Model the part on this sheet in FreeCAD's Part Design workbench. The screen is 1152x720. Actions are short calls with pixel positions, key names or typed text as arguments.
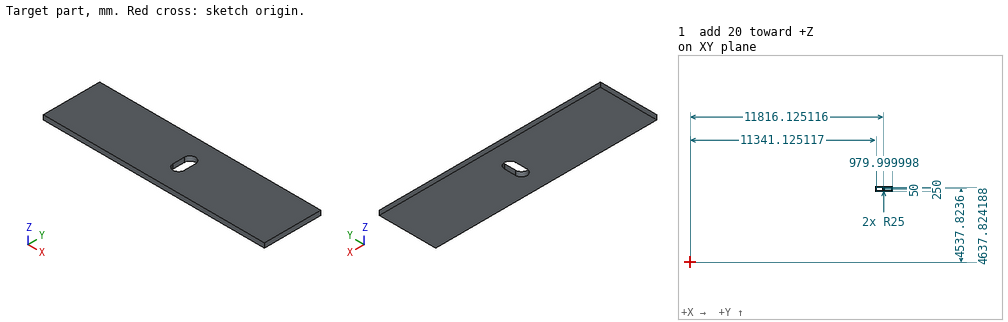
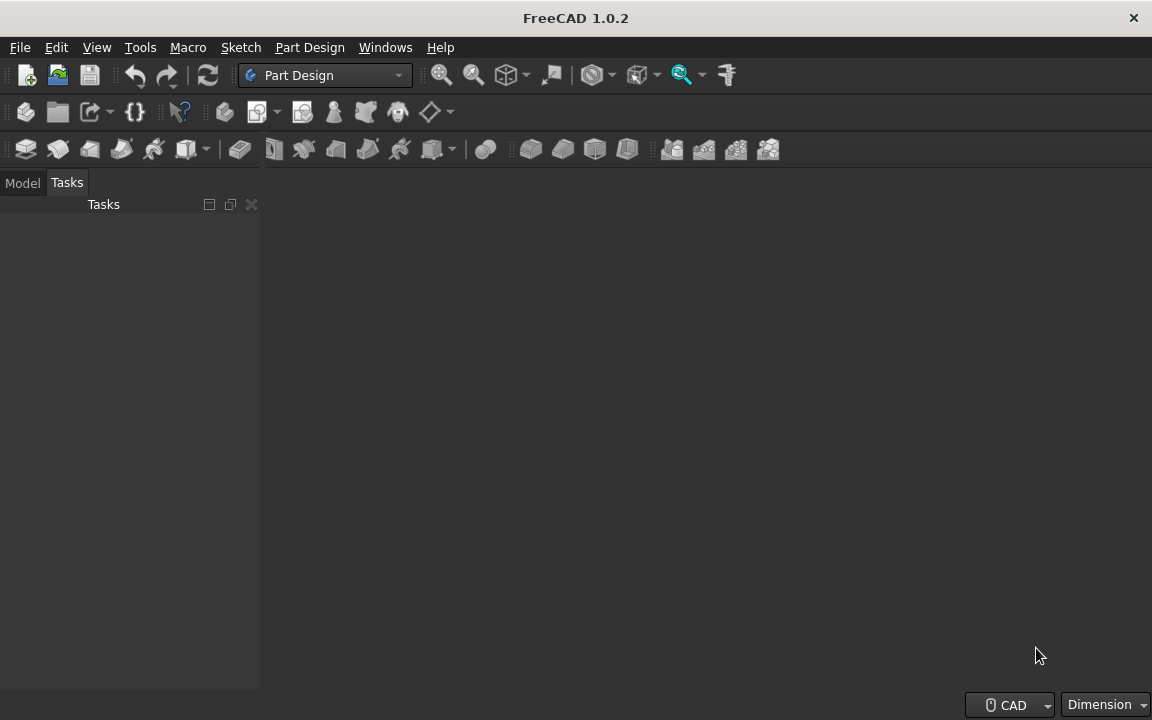
key(ctrl+n)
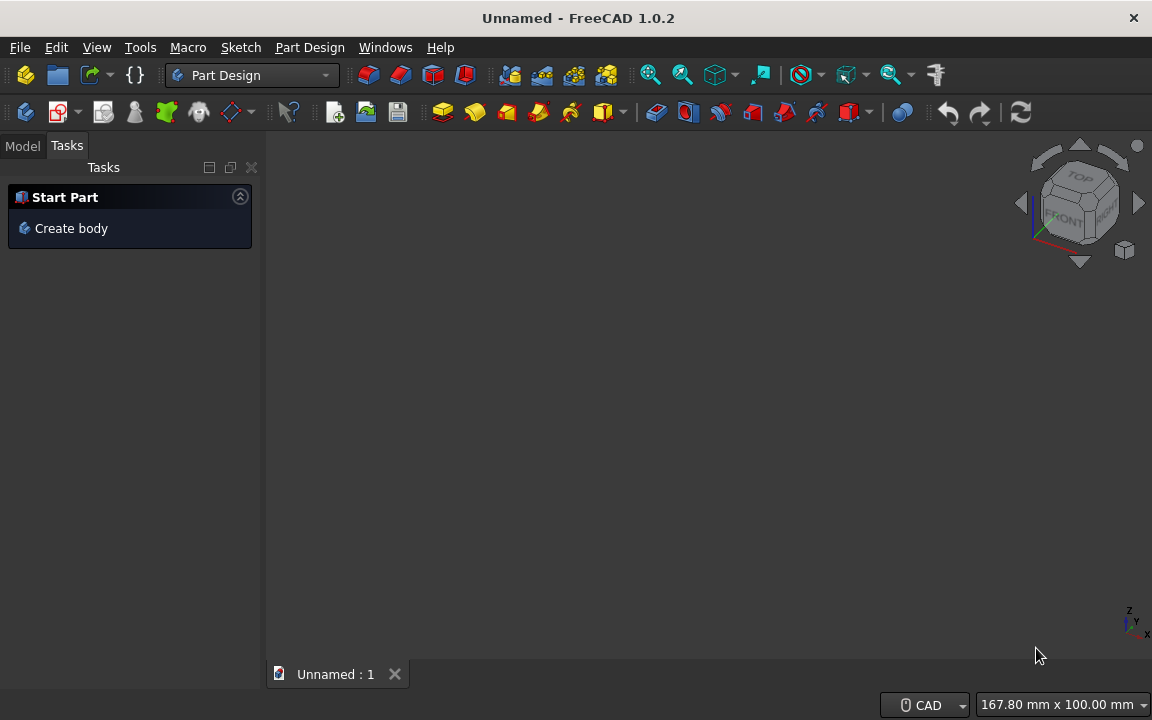
click(58, 112)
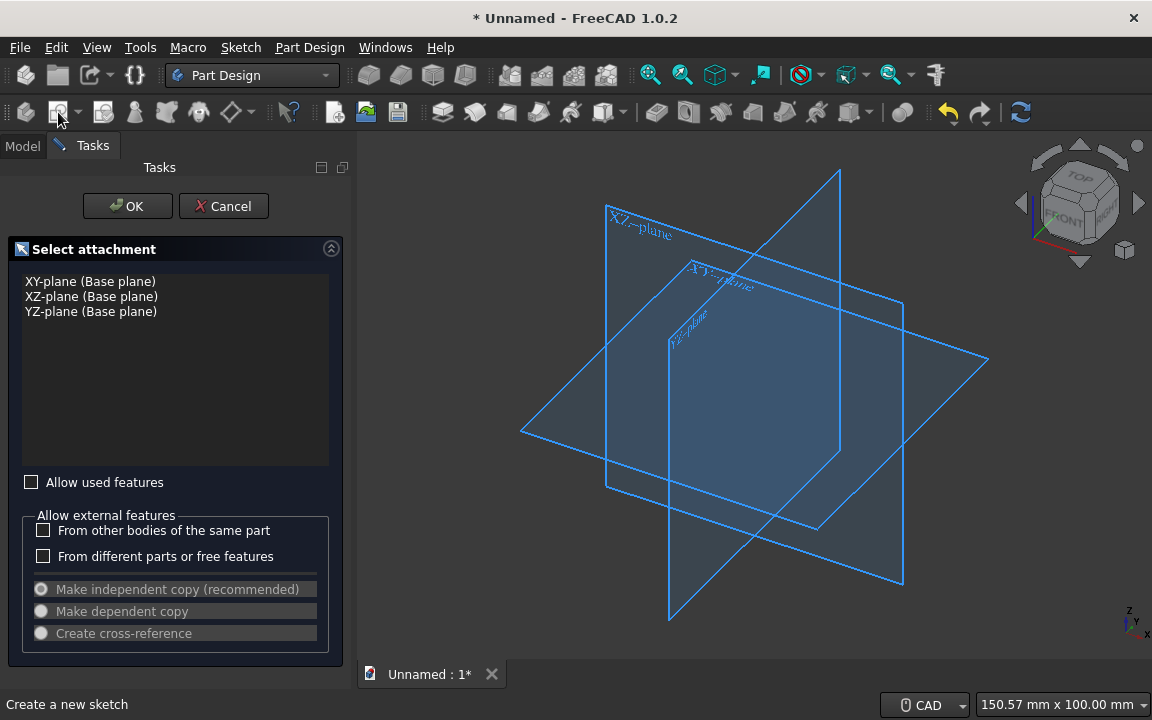
click(82, 282)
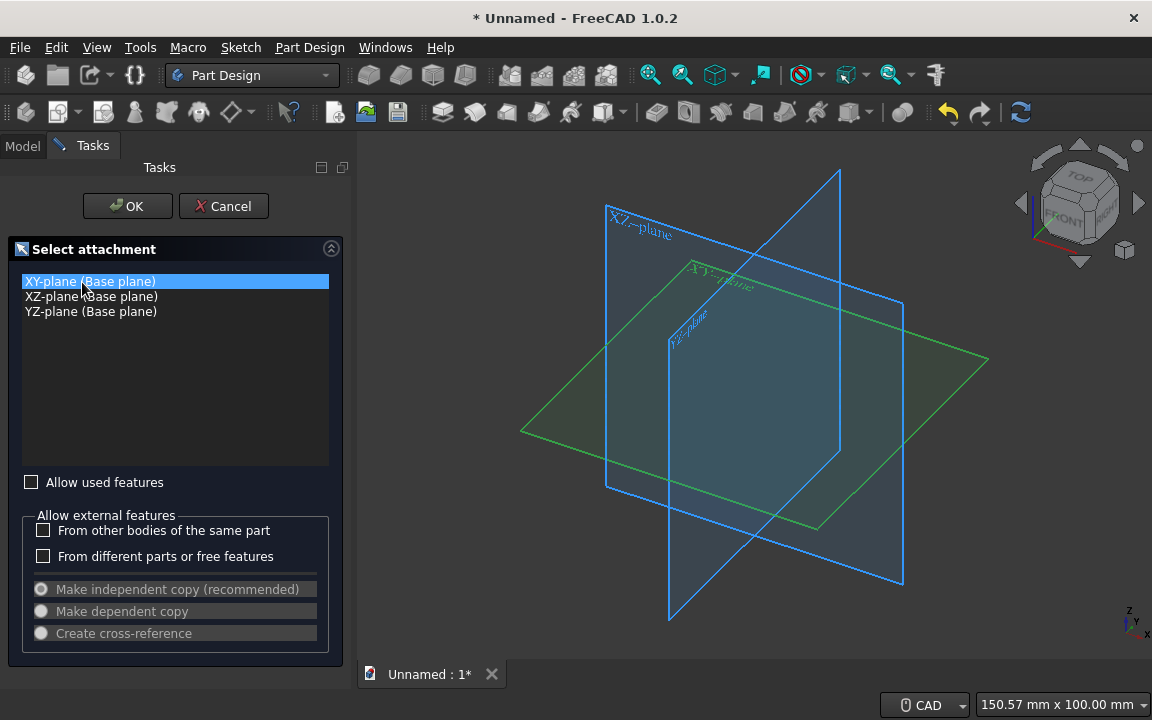
click(128, 206)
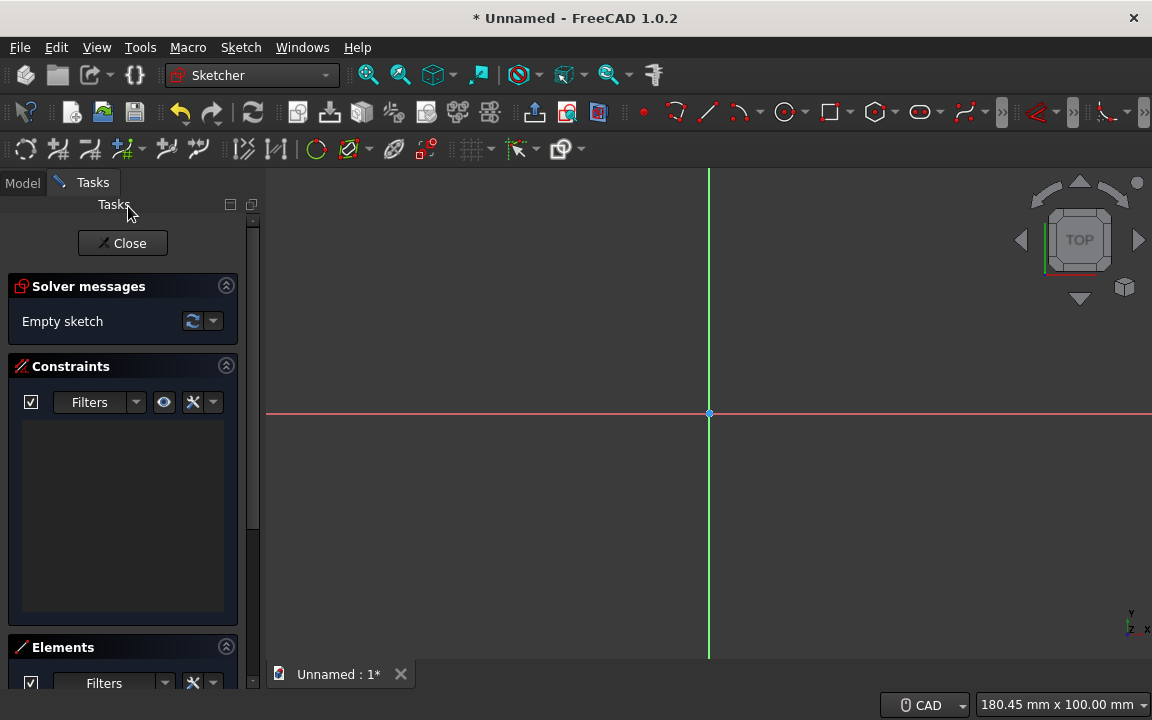
scroll(640, 414, down, 11)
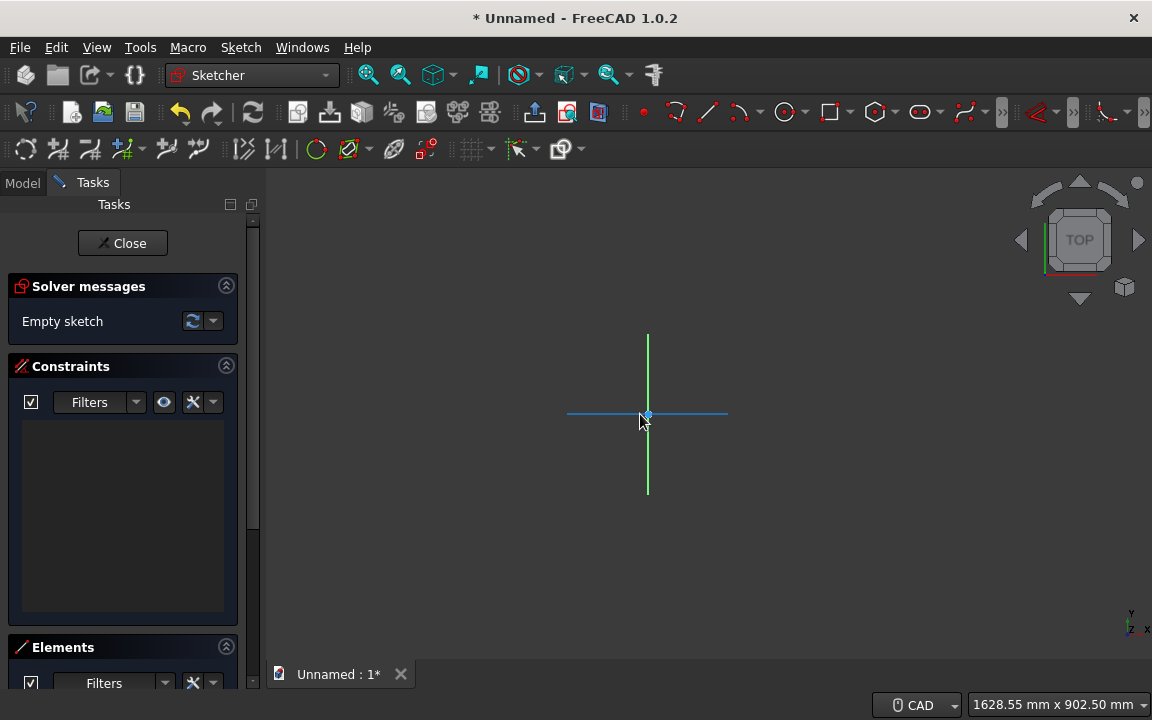
scroll(640, 414, down, 5)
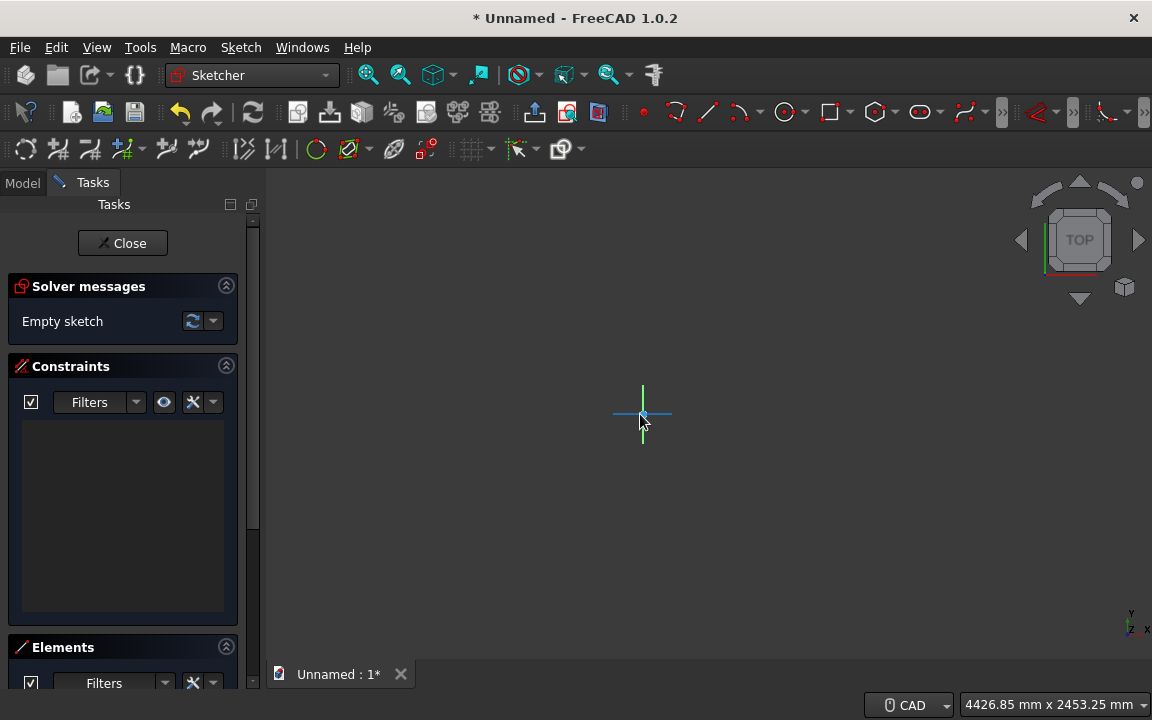
scroll(640, 414, down, 5)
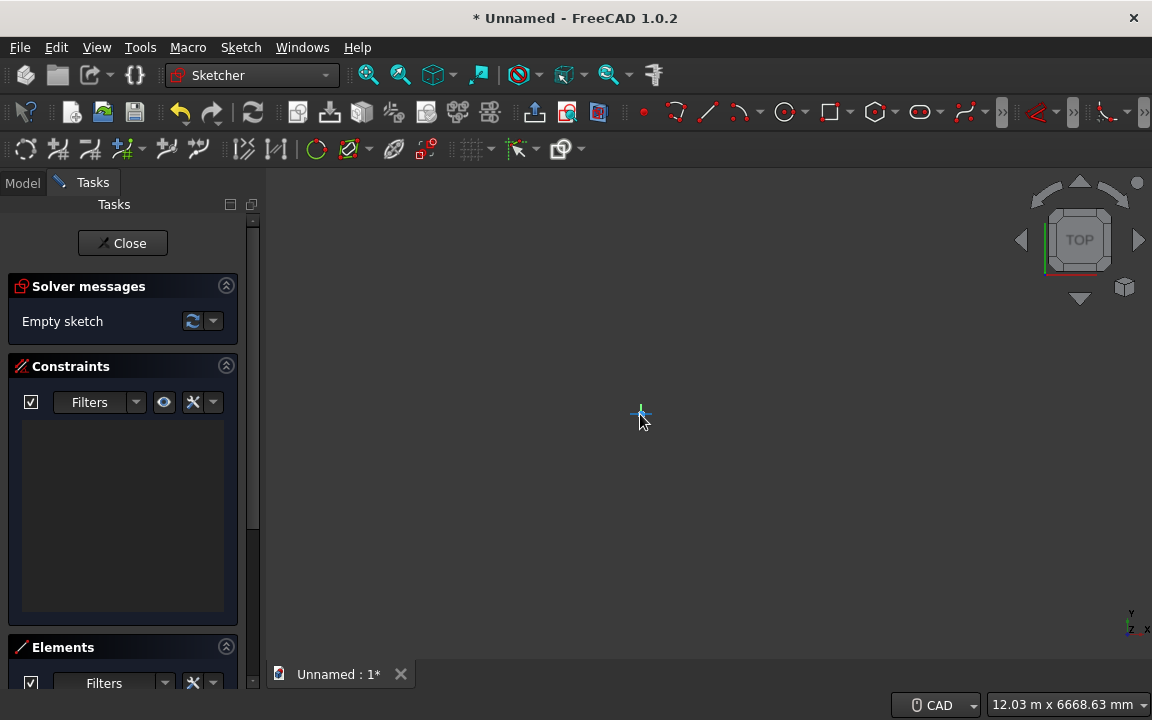
scroll(640, 414, down, 5)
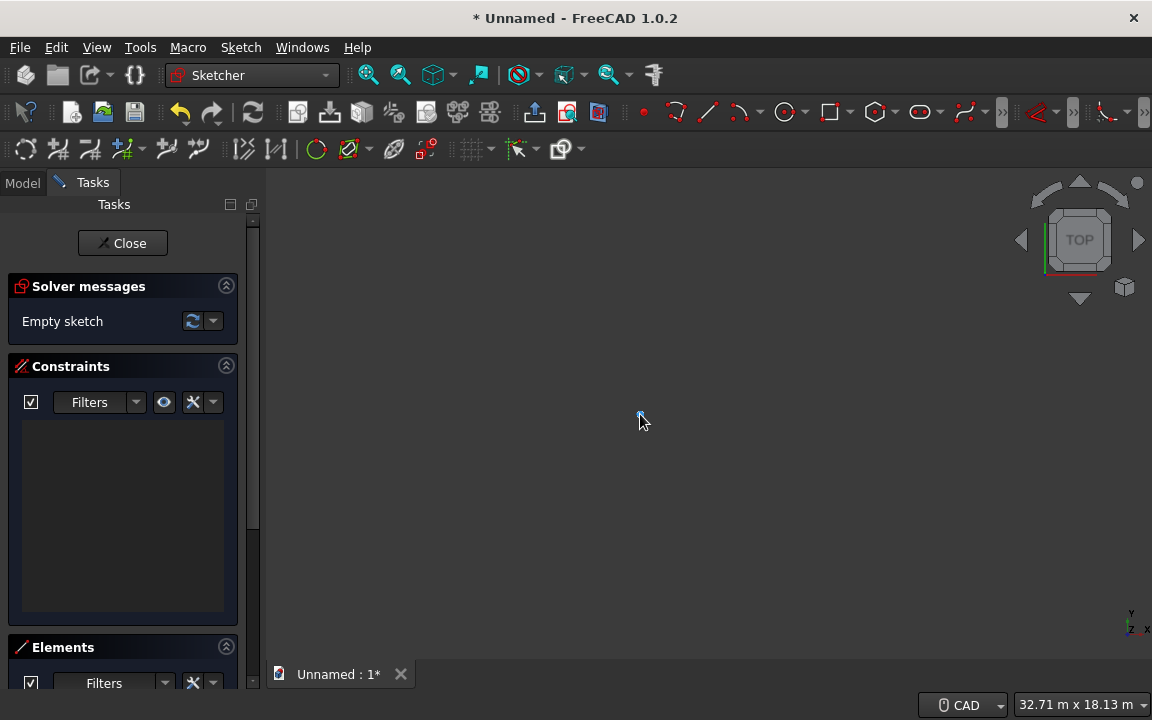
scroll(978, 286, up, 15)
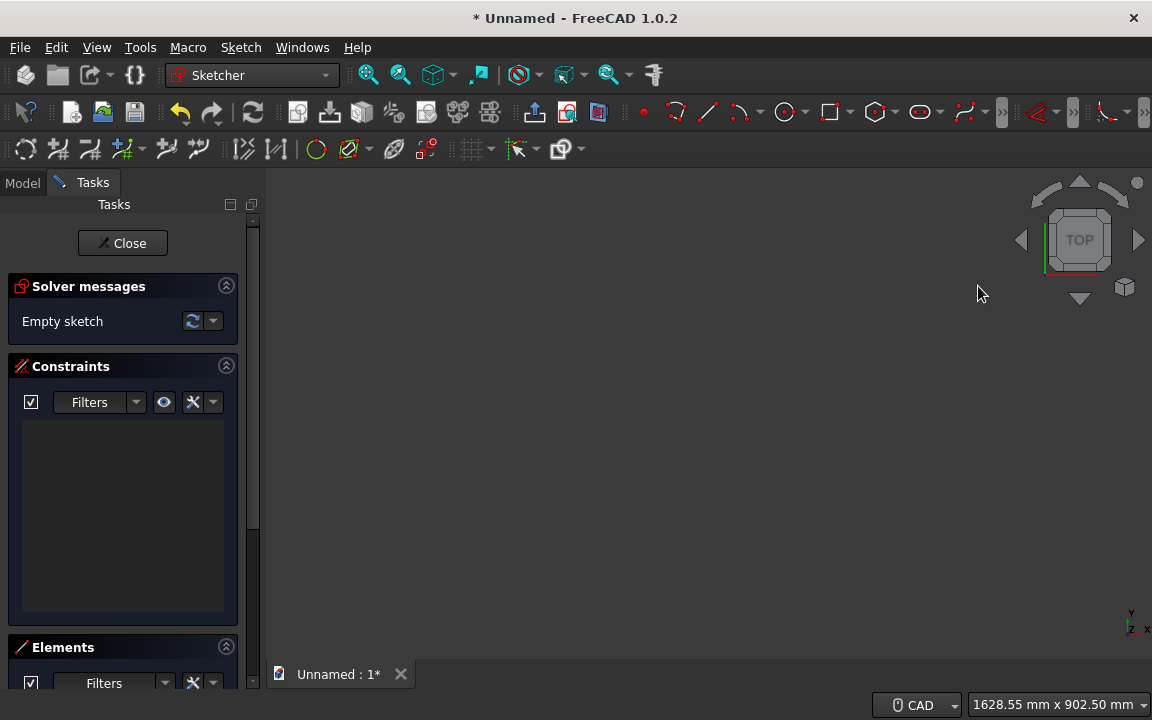
key(g)
key(r)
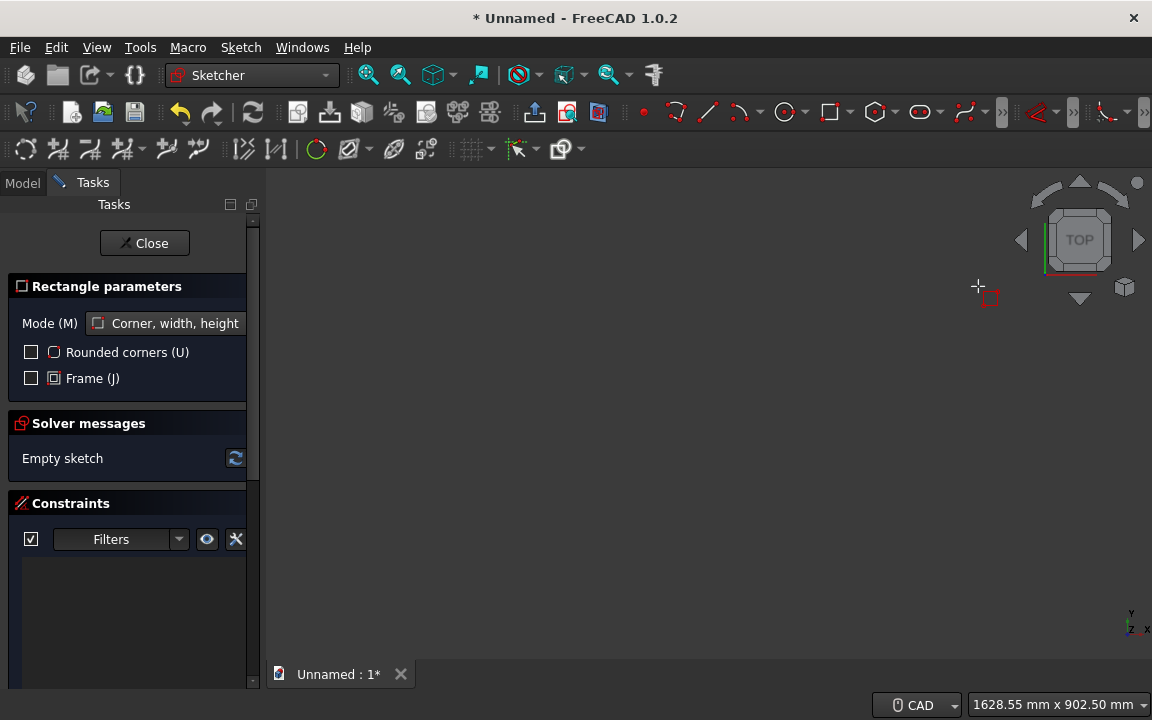
click(360, 339)
click(893, 475)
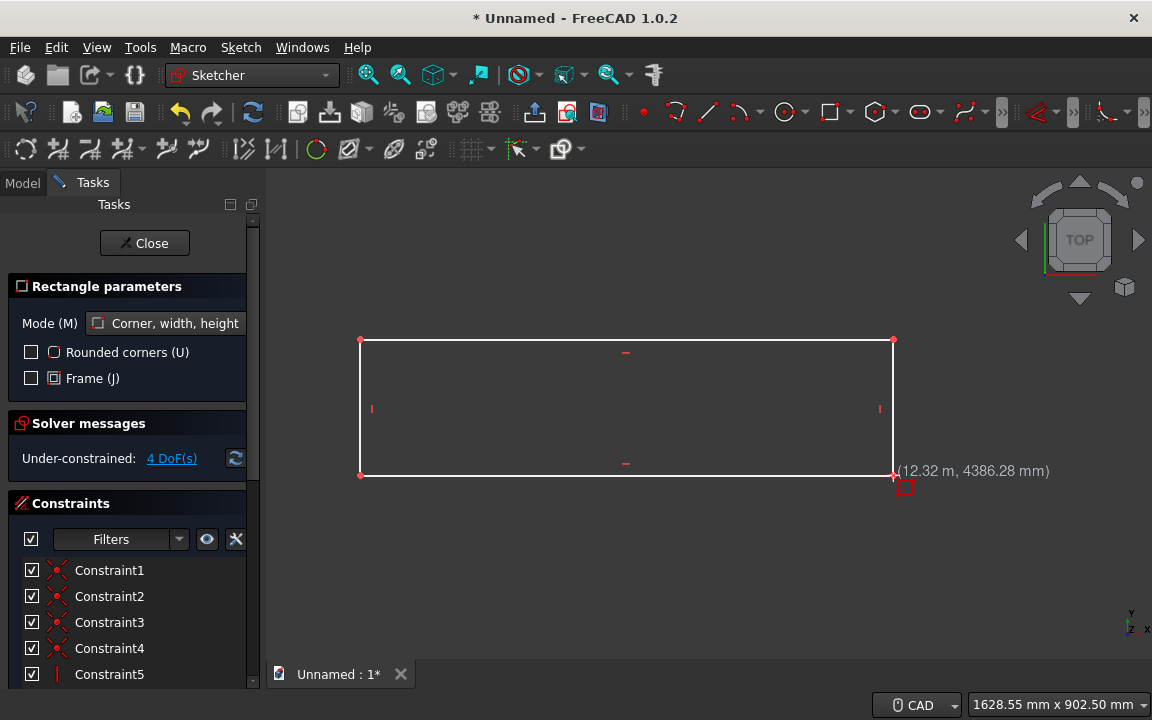
click(708, 112)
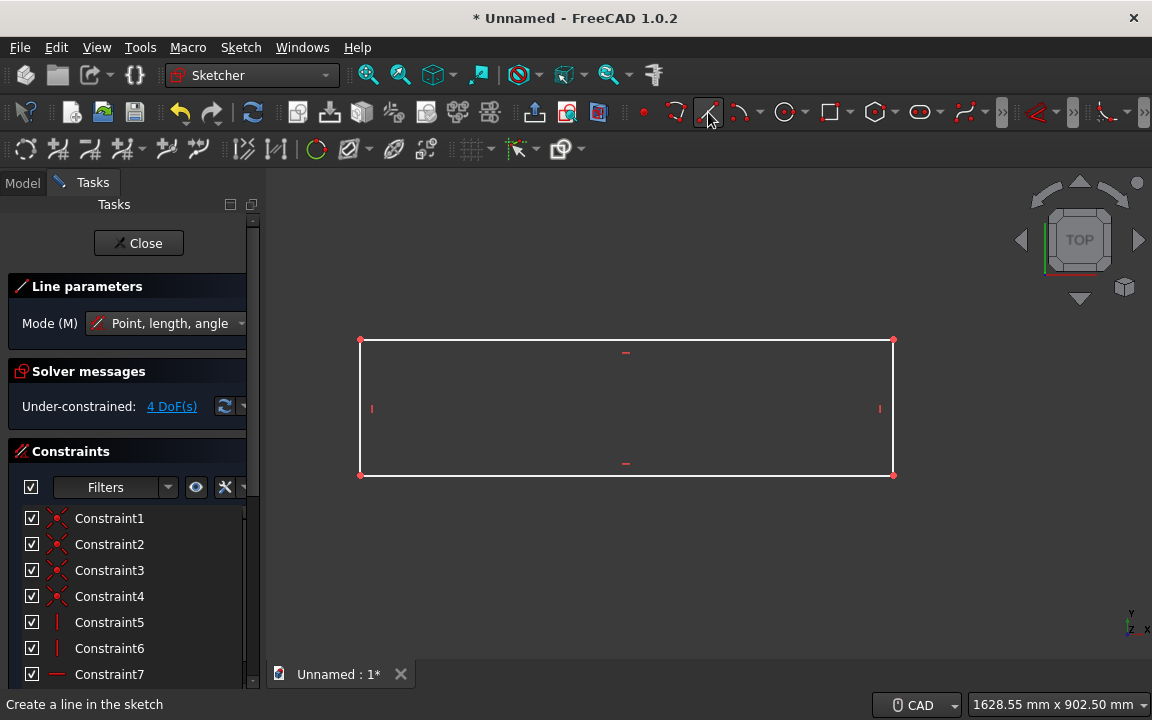
click(618, 421)
click(618, 394)